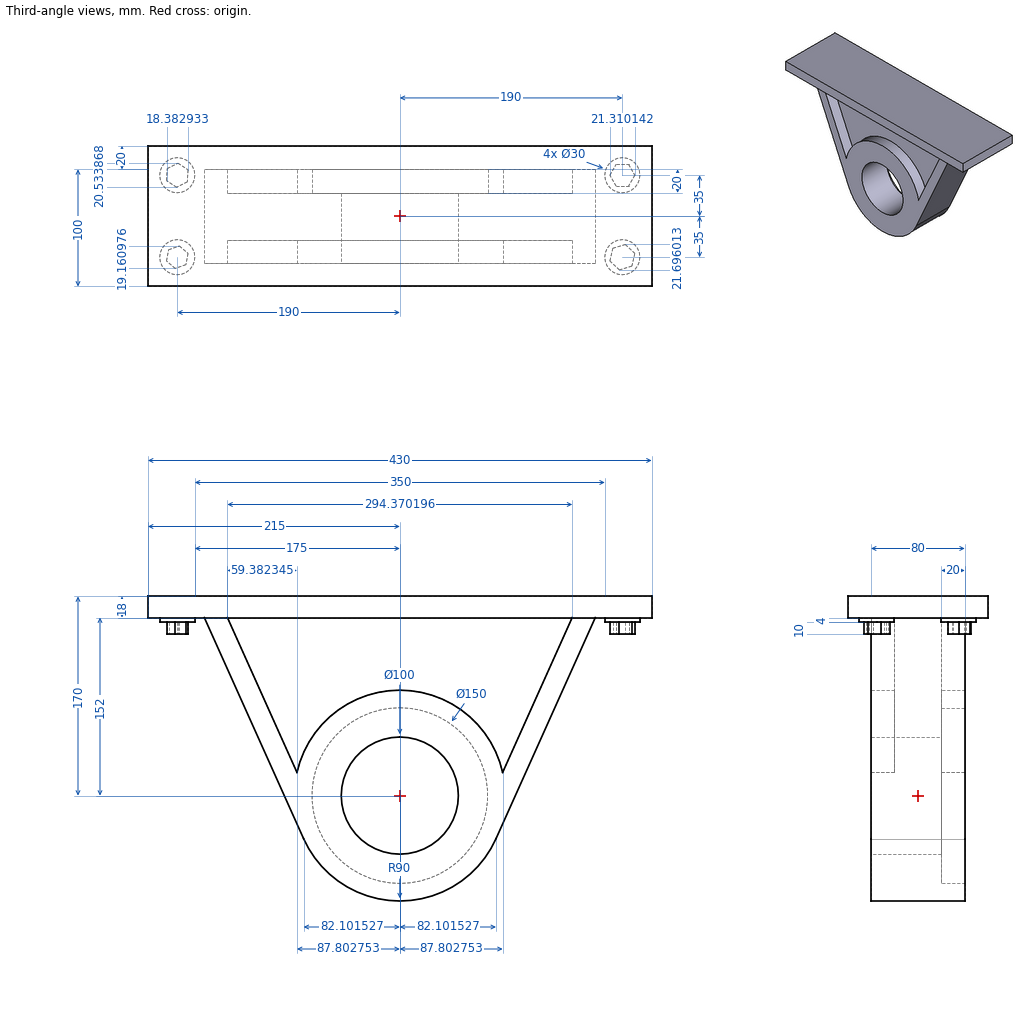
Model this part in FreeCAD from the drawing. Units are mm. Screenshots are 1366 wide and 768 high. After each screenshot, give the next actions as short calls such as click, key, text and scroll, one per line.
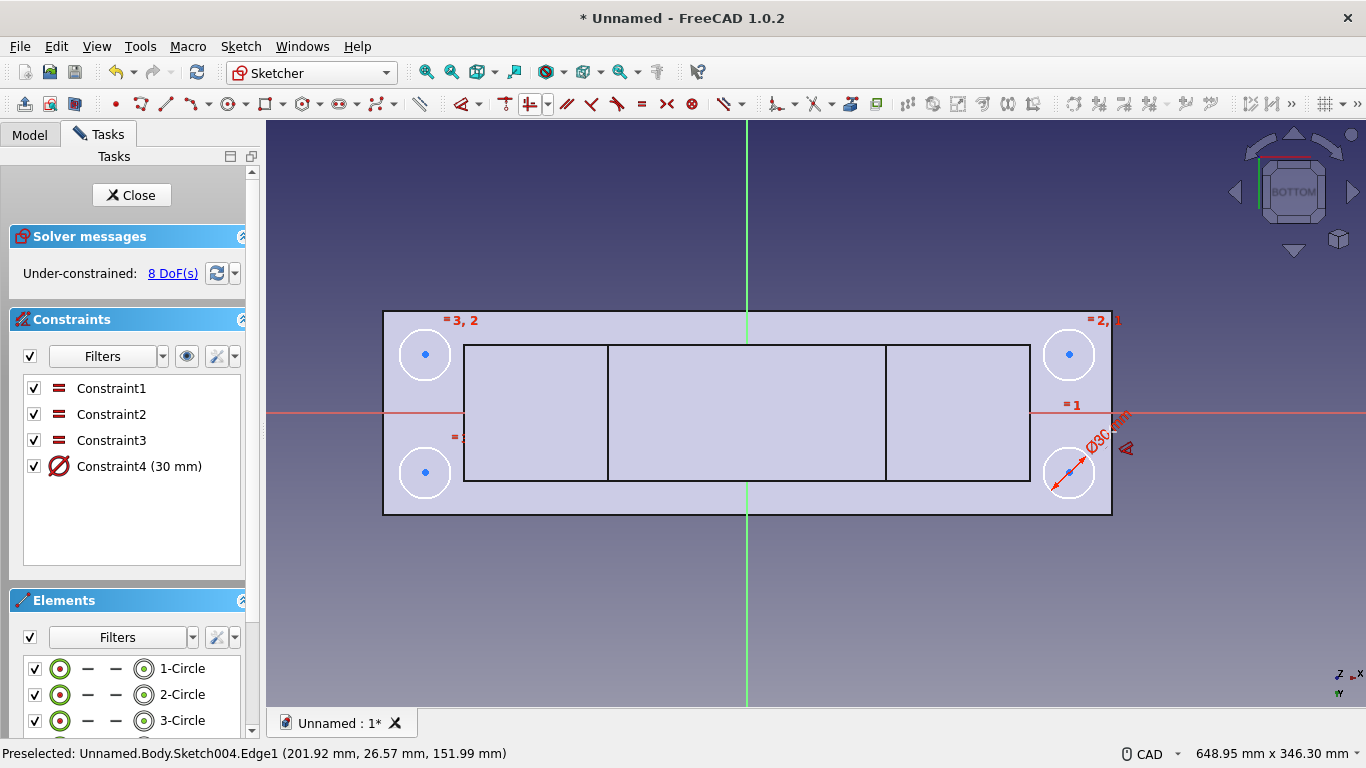
click(1069, 473)
click(713, 443)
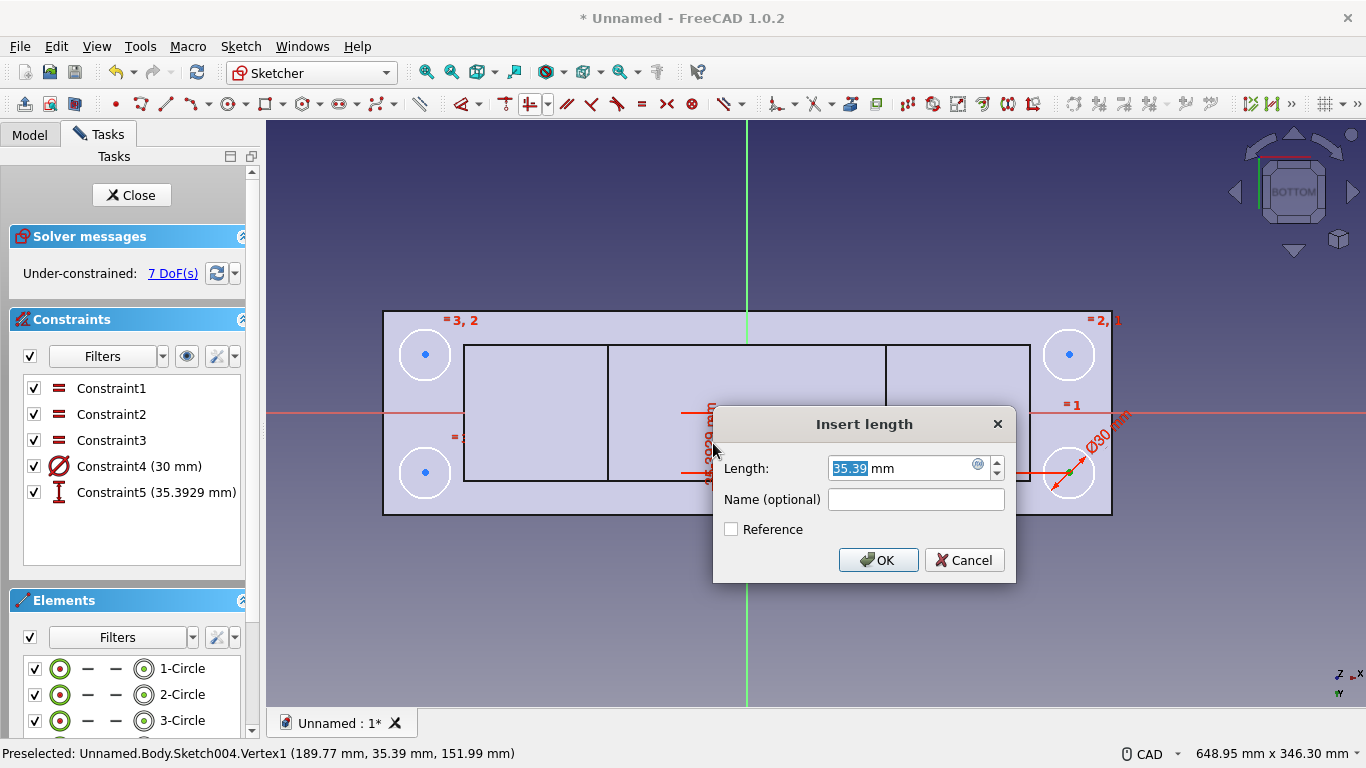
text(35)
key(Return)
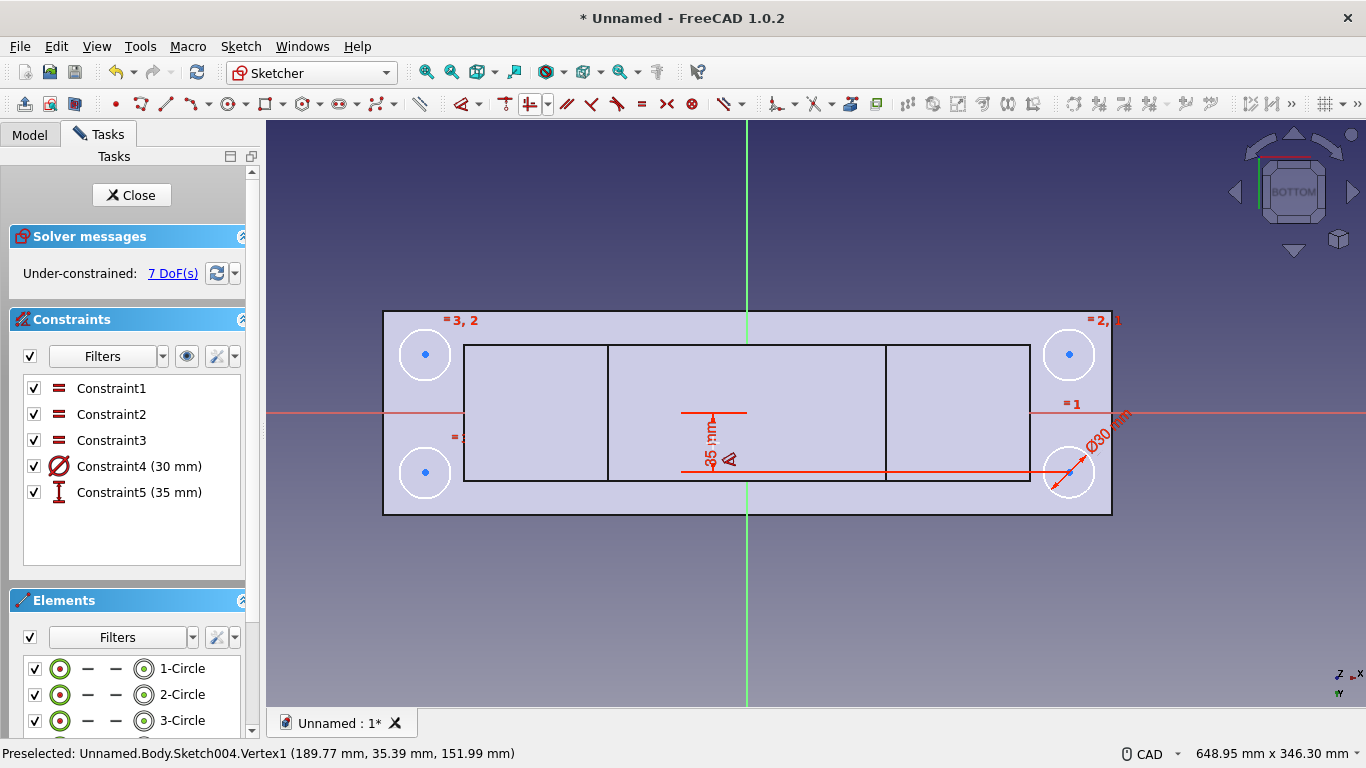
click(1069, 355)
click(1103, 384)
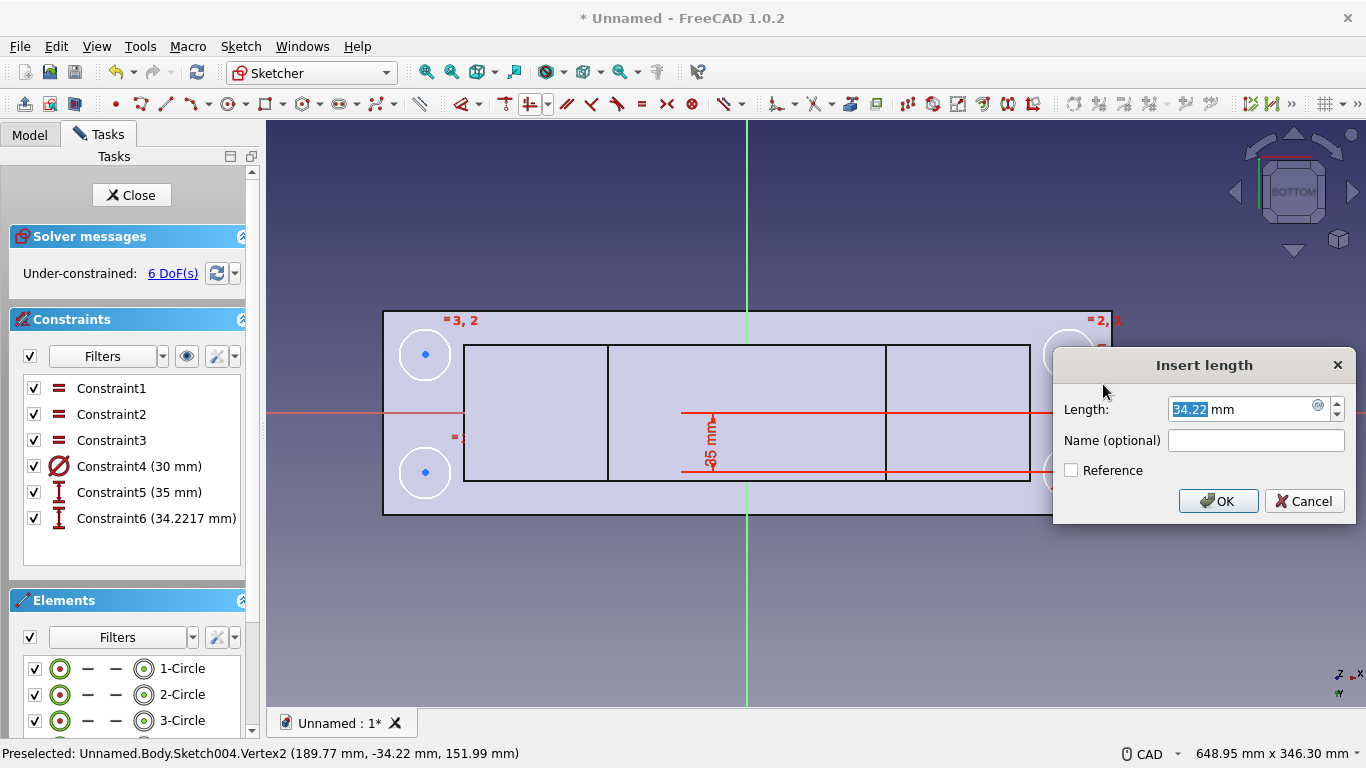
text(35)
key(Return)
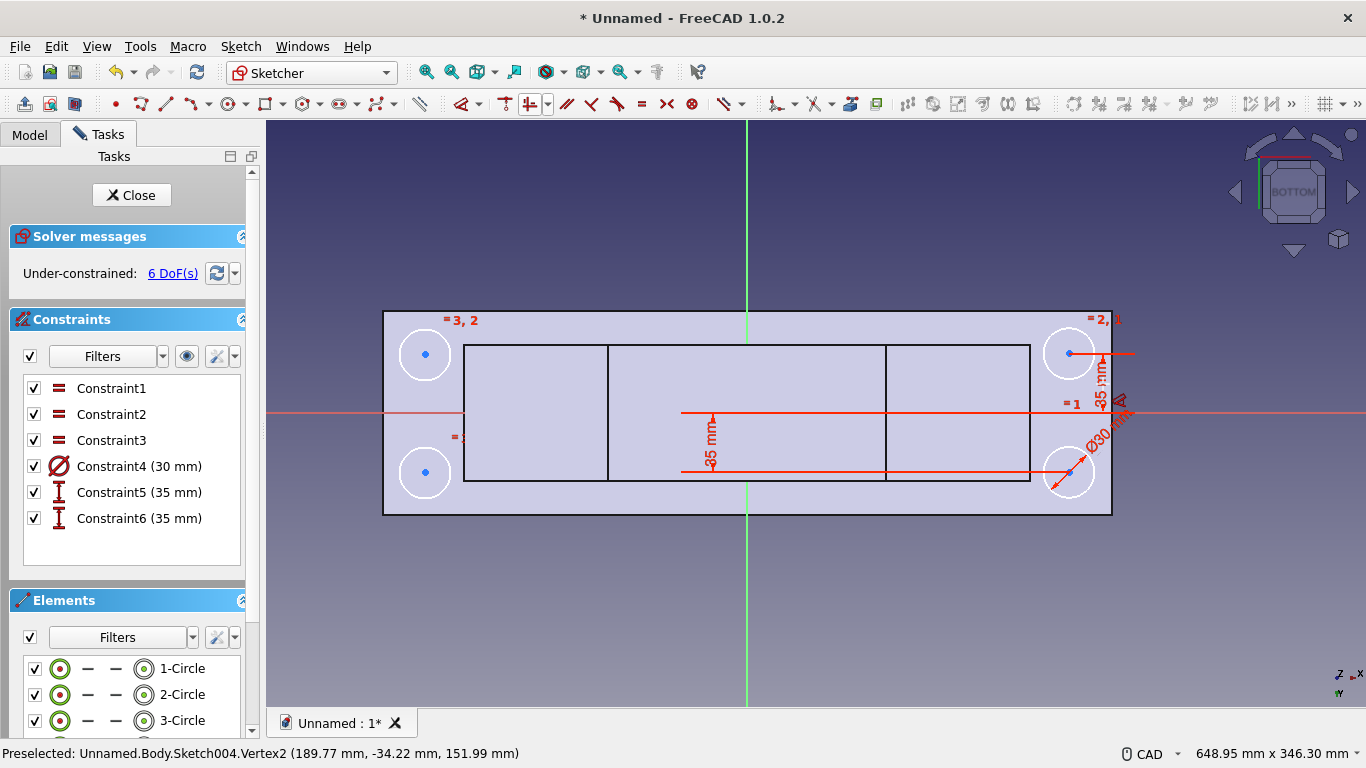
click(425, 355)
click(391, 384)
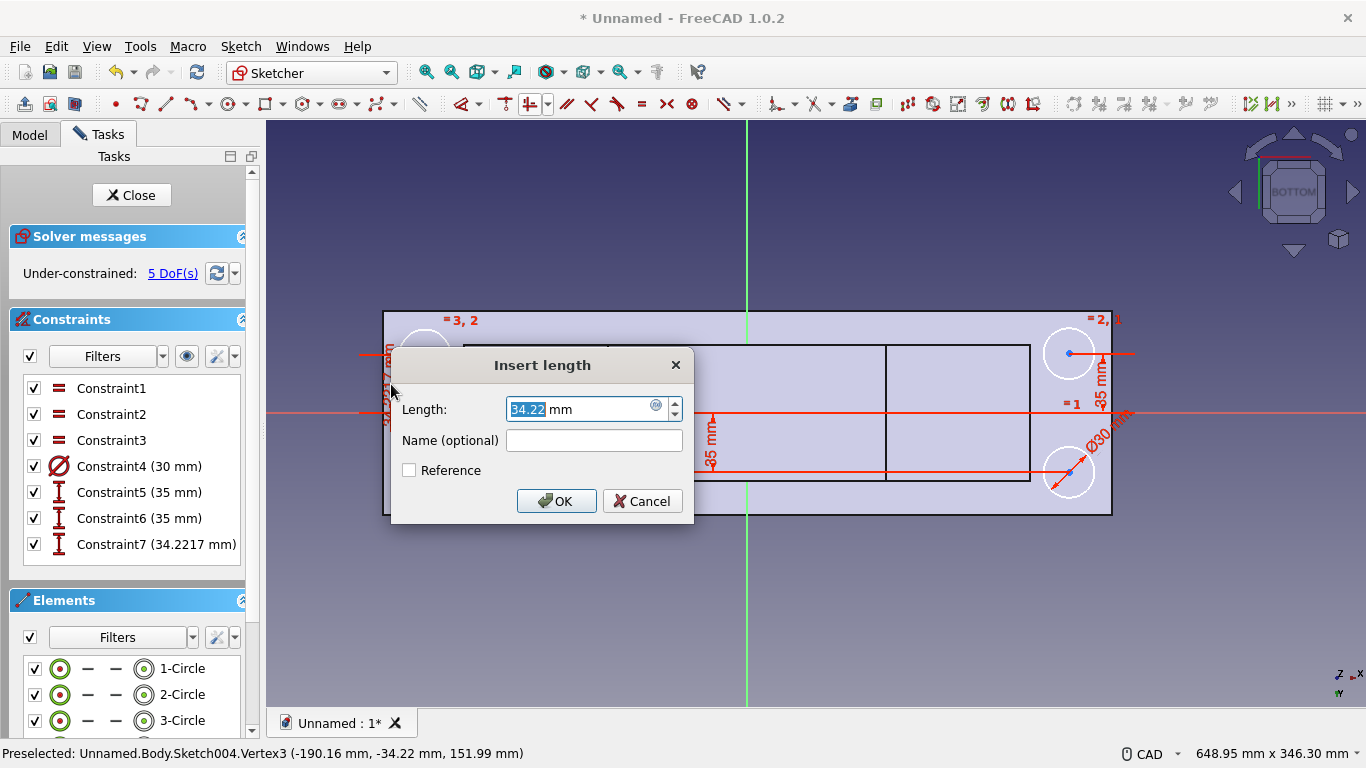
text(35)
key(Return)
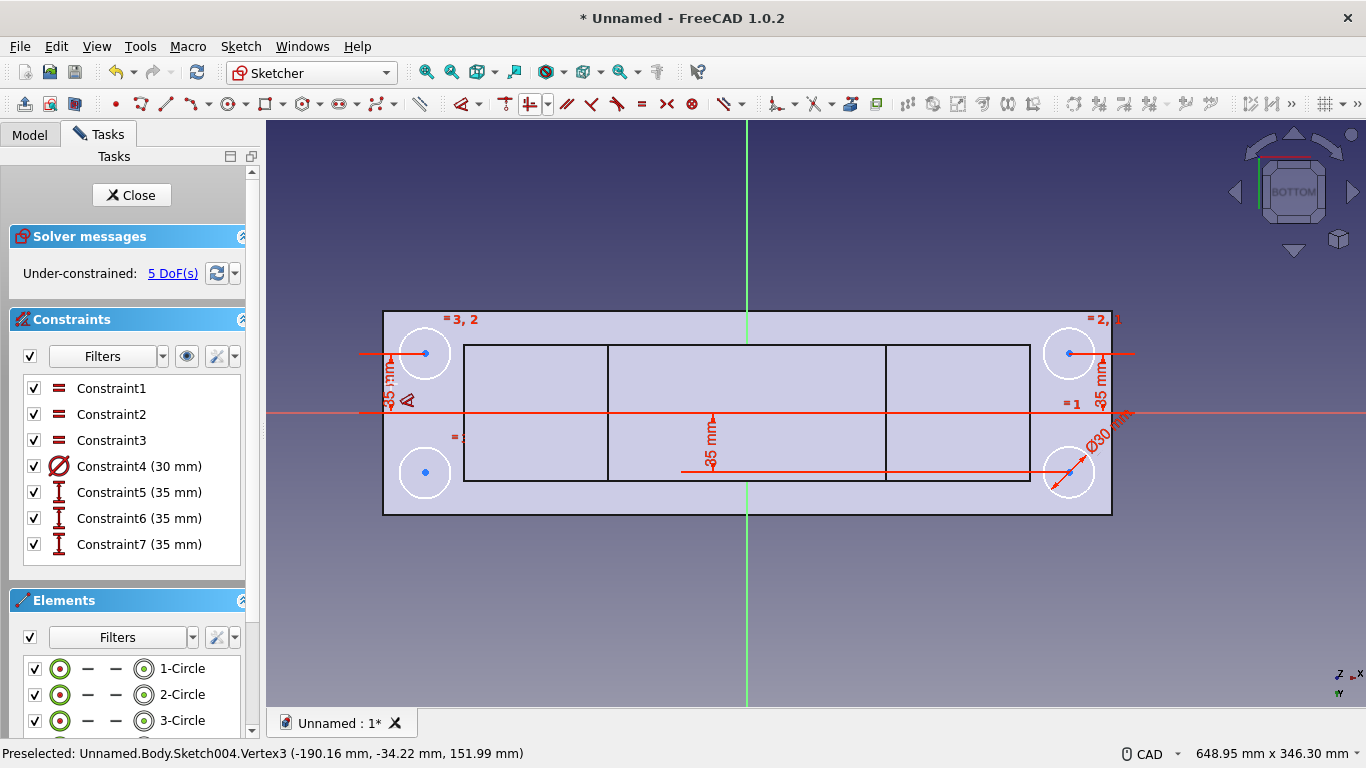
click(425, 473)
click(391, 443)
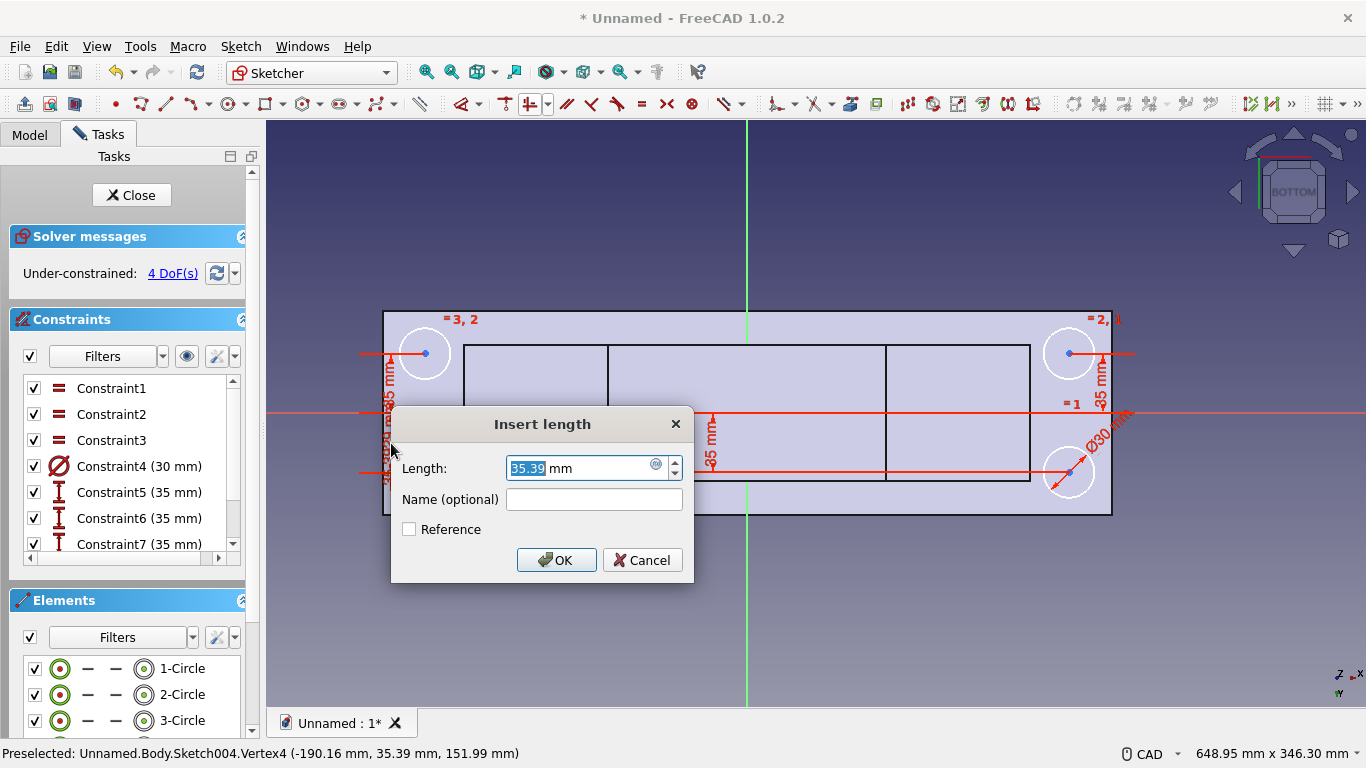
text(35)
key(Return)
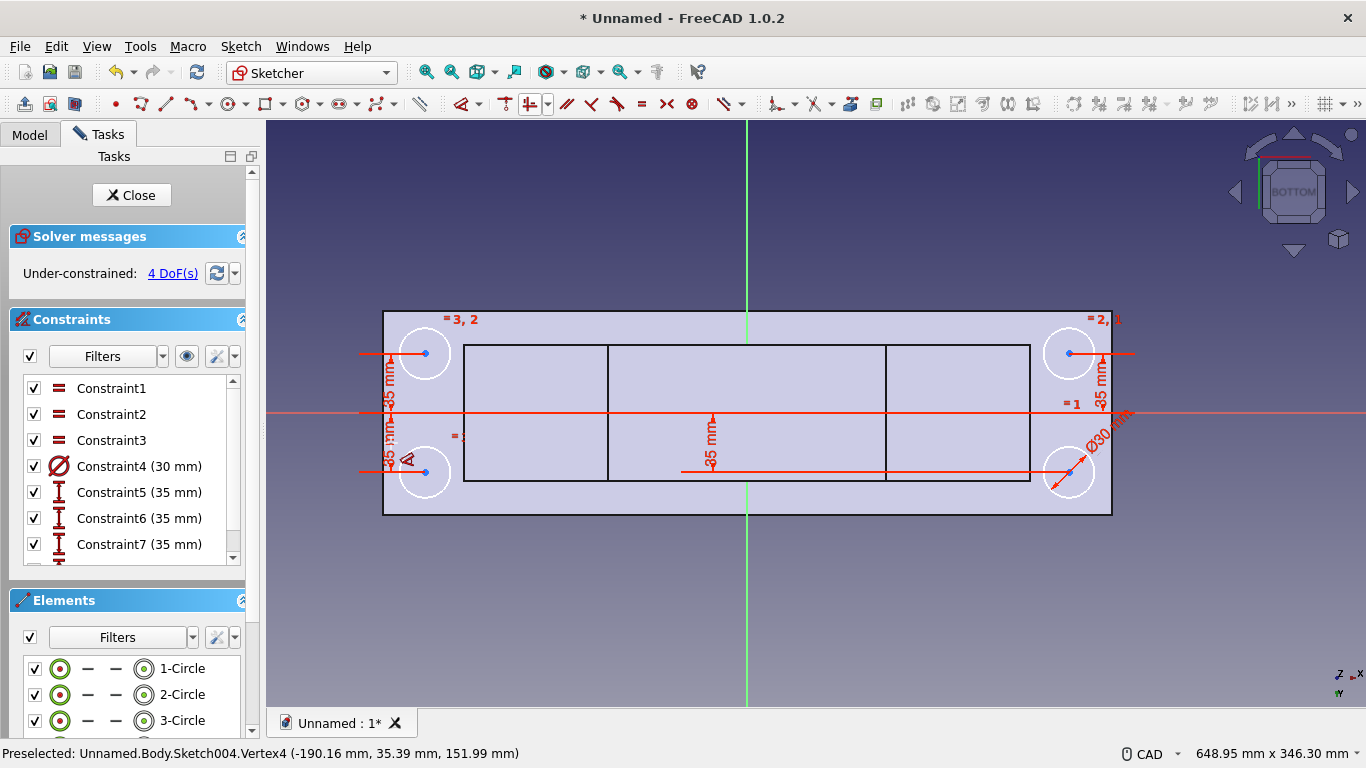
click(1069, 472)
click(908, 506)